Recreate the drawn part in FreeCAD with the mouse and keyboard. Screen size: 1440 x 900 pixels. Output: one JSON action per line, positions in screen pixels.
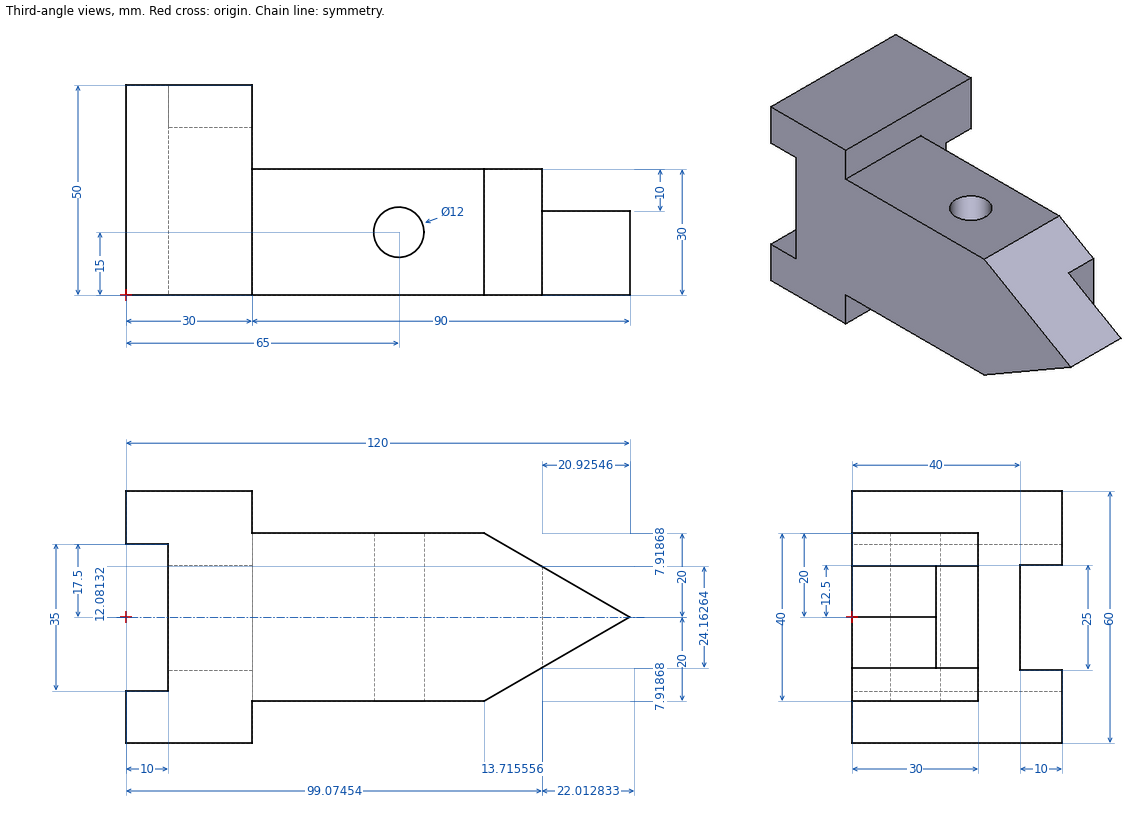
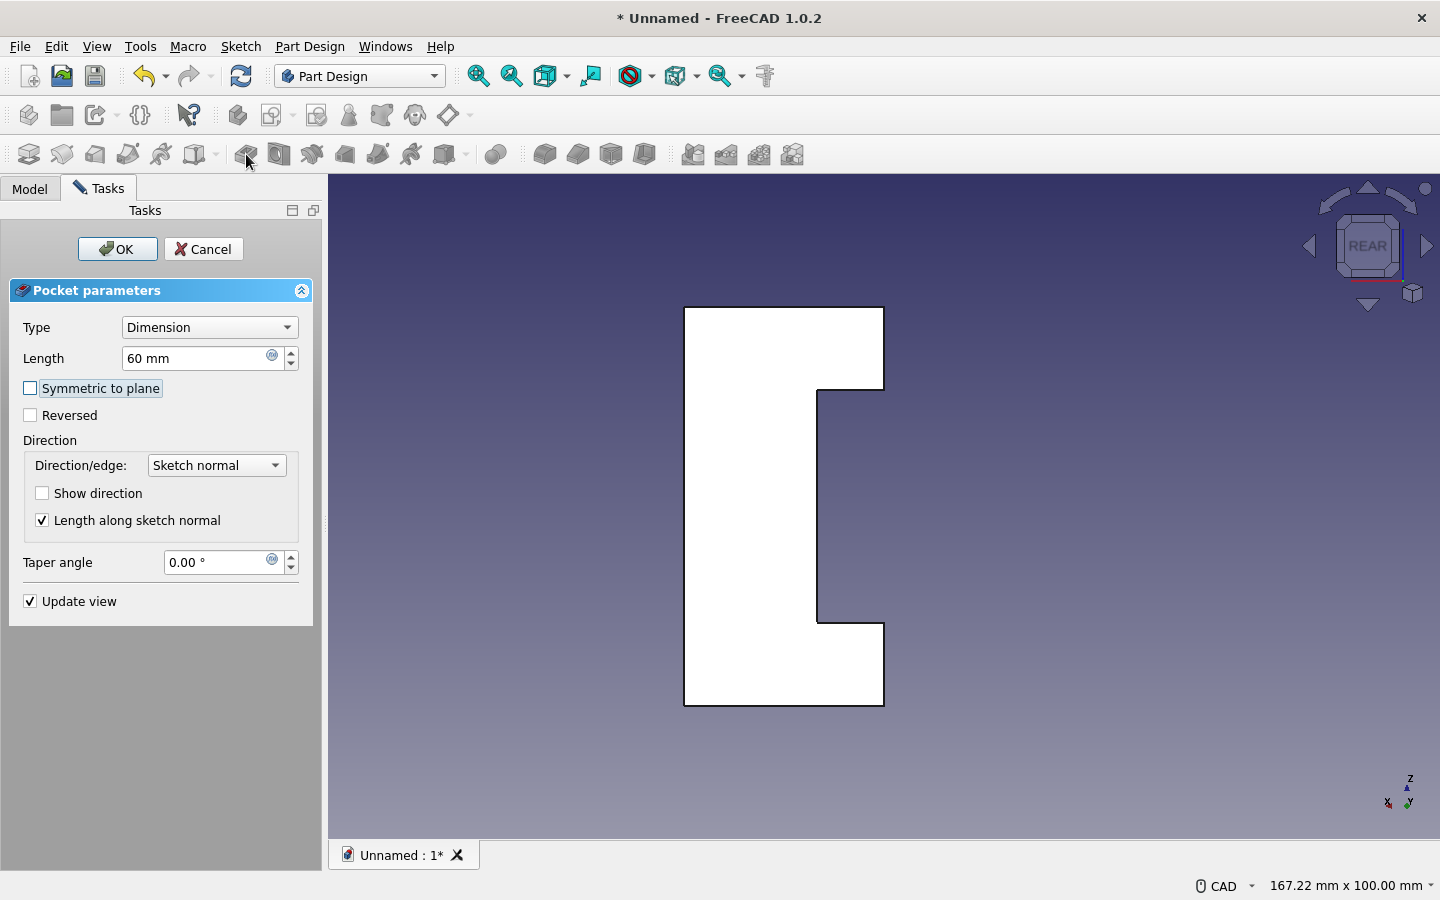
{"action": "left_click", "coordinate": [118, 249]}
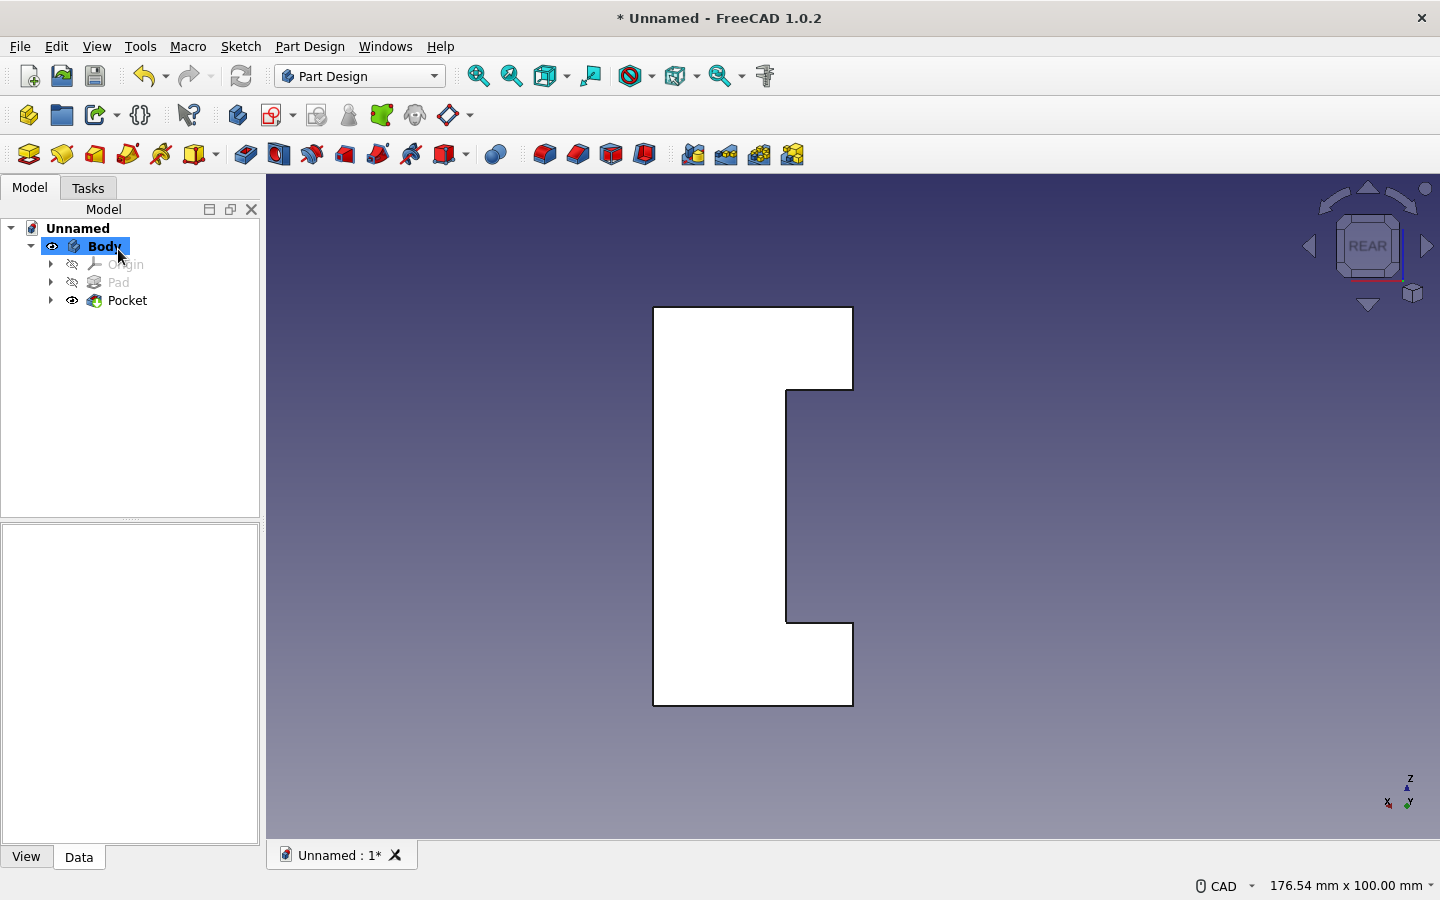
{"action": "key", "text": "0"}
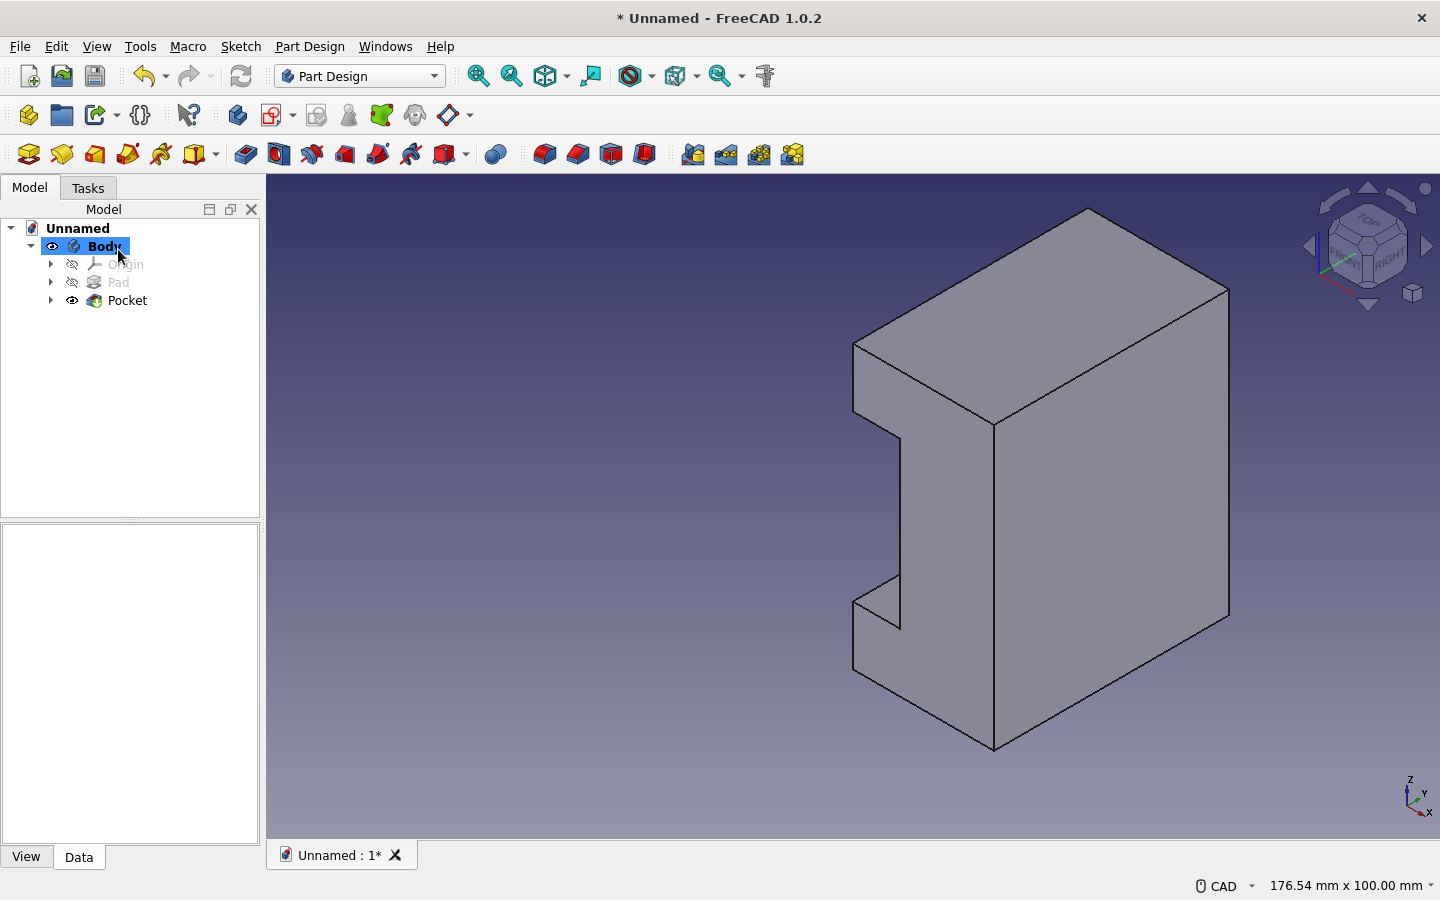
{"action": "left_click", "coordinate": [1112, 519]}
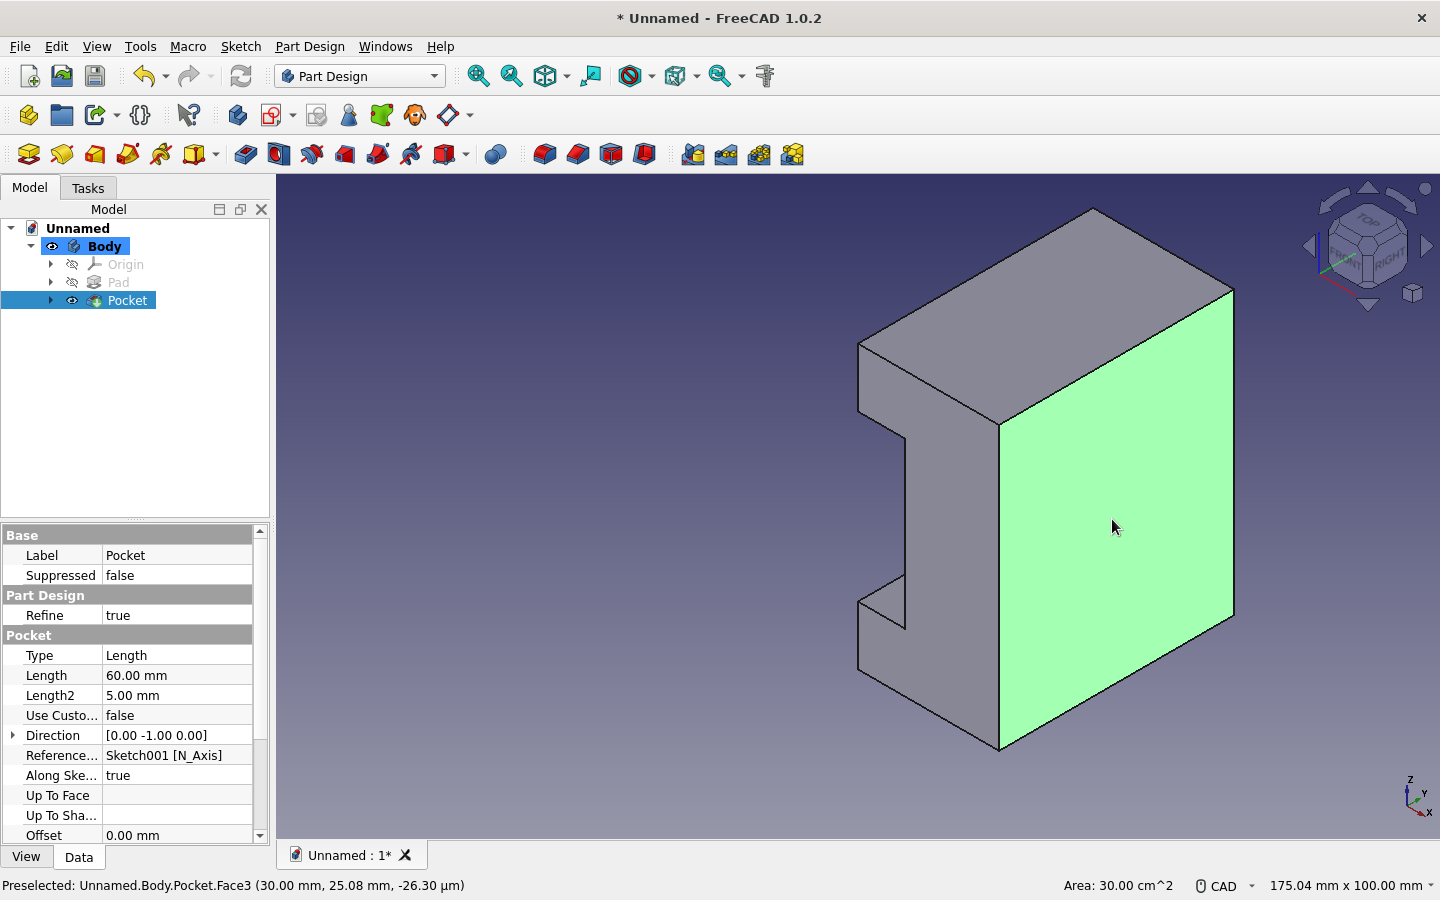
{"action": "left_click", "coordinate": [270, 116]}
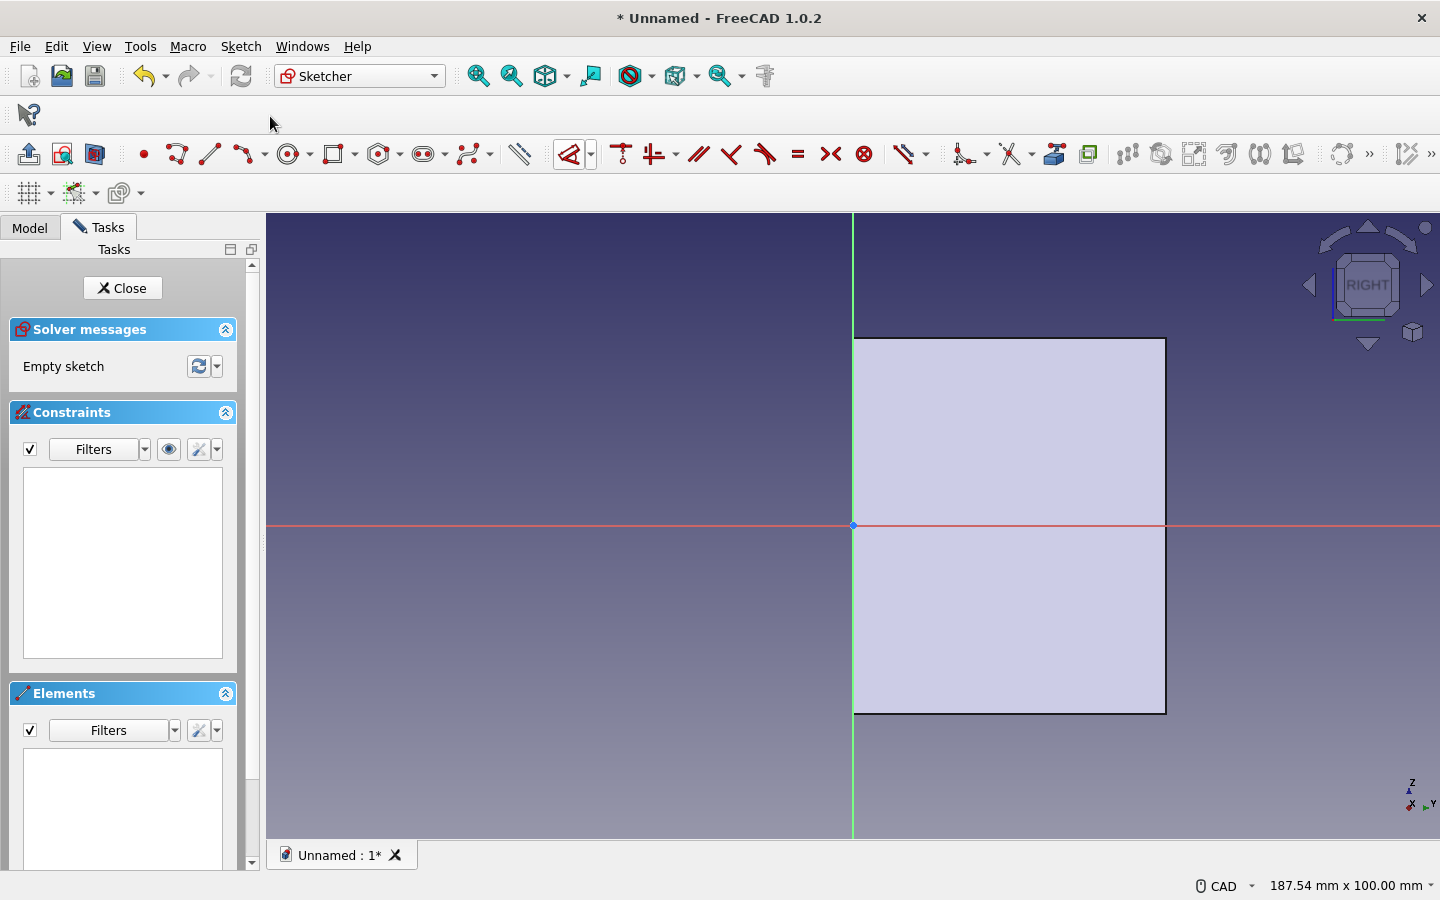
{"action": "scroll", "coordinate": [1193, 526], "scroll_direction": "up", "scroll_amount": 4}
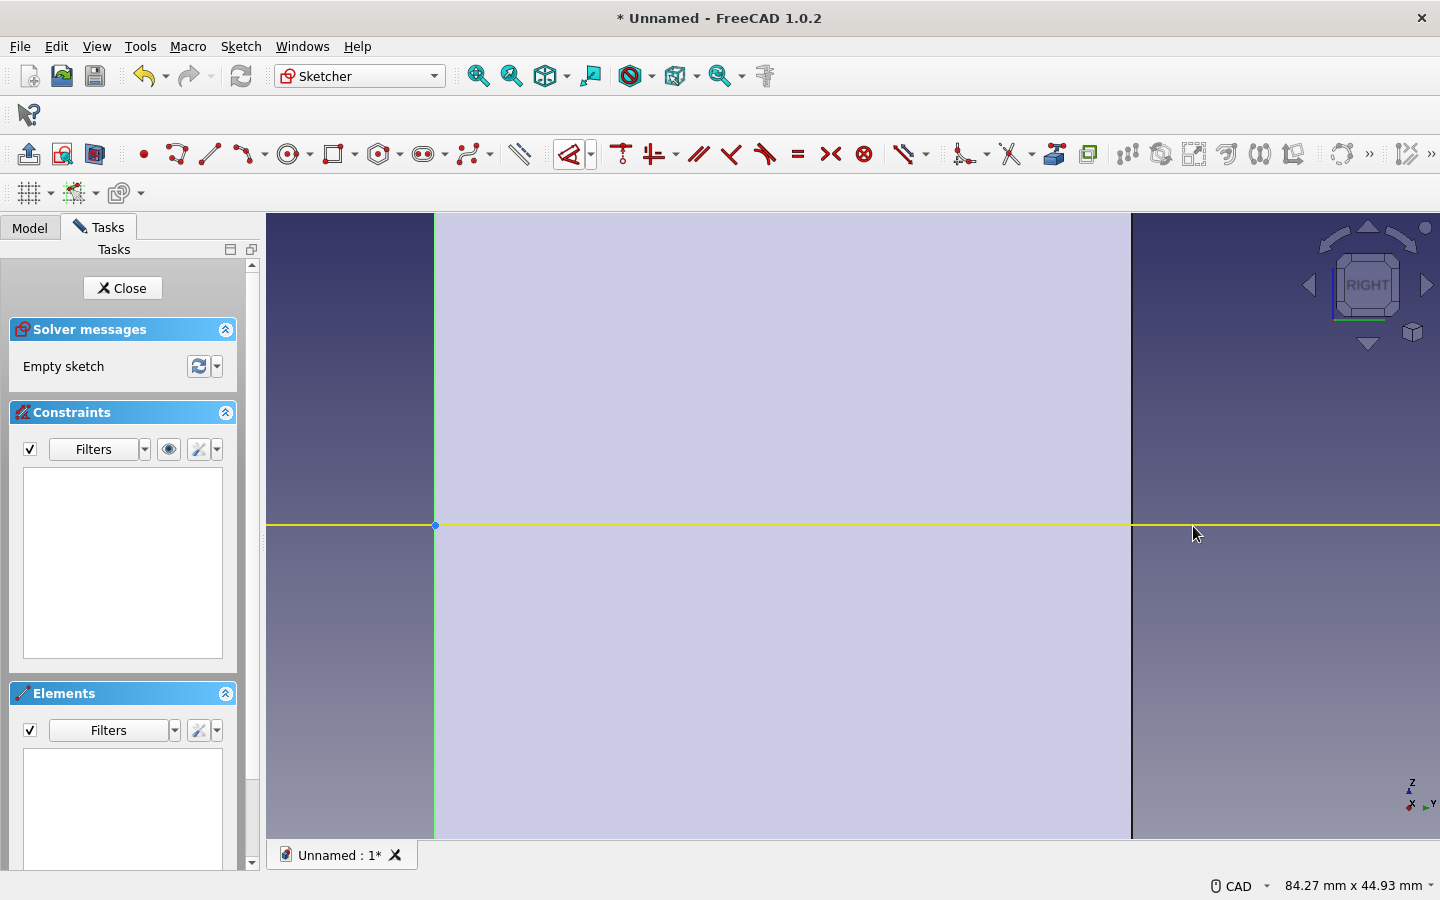
{"action": "left_click", "coordinate": [332, 154]}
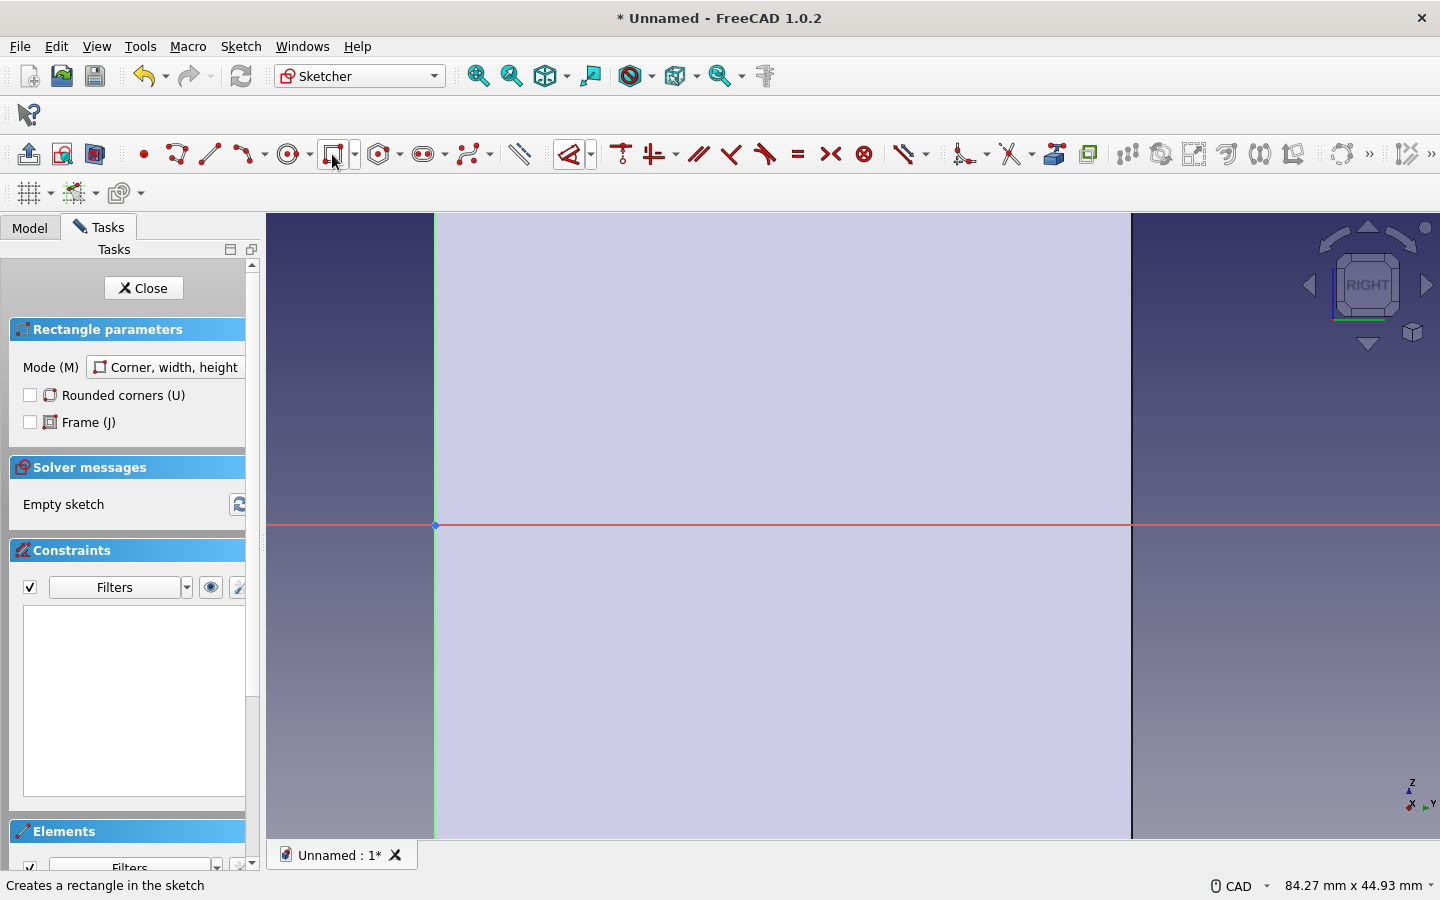
{"action": "left_click", "coordinate": [993, 351]}
{"action": "left_click", "coordinate": [1132, 700]}
{"action": "key", "text": "Escape"}